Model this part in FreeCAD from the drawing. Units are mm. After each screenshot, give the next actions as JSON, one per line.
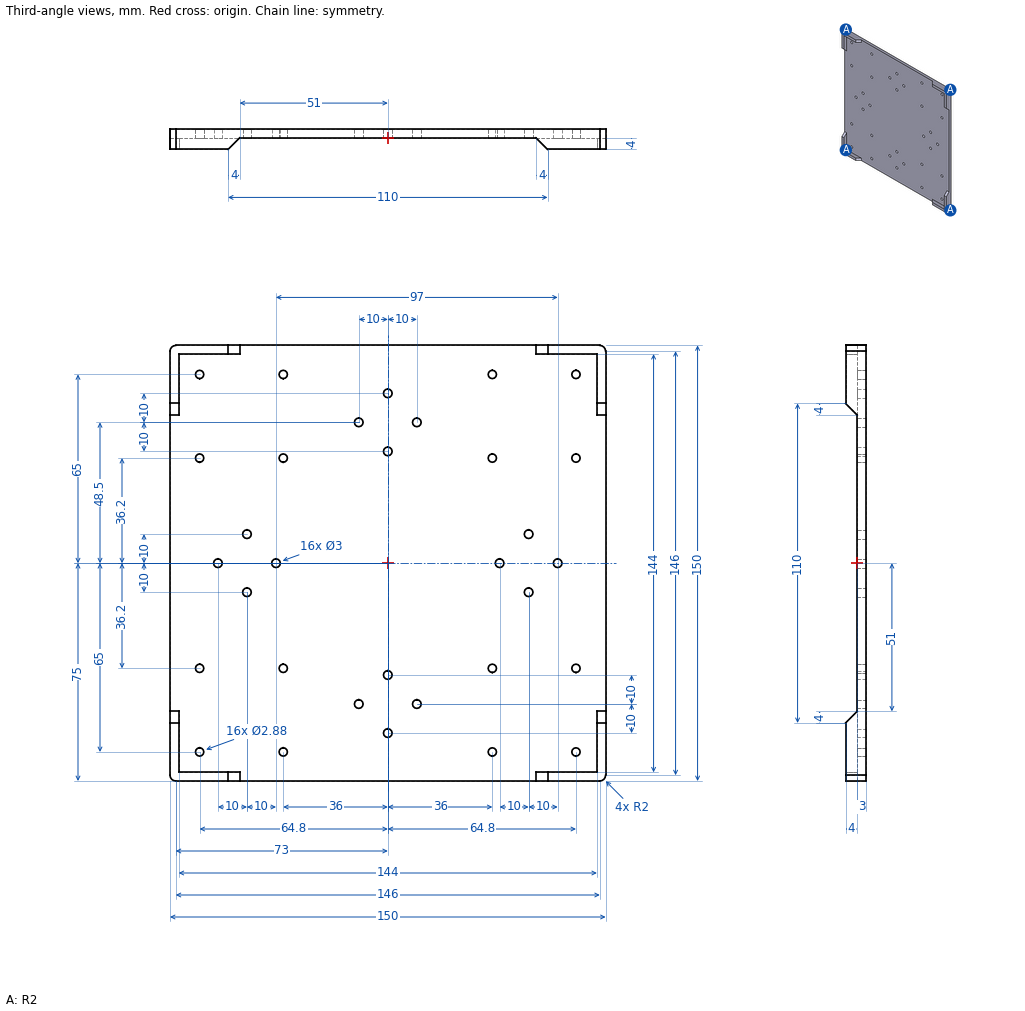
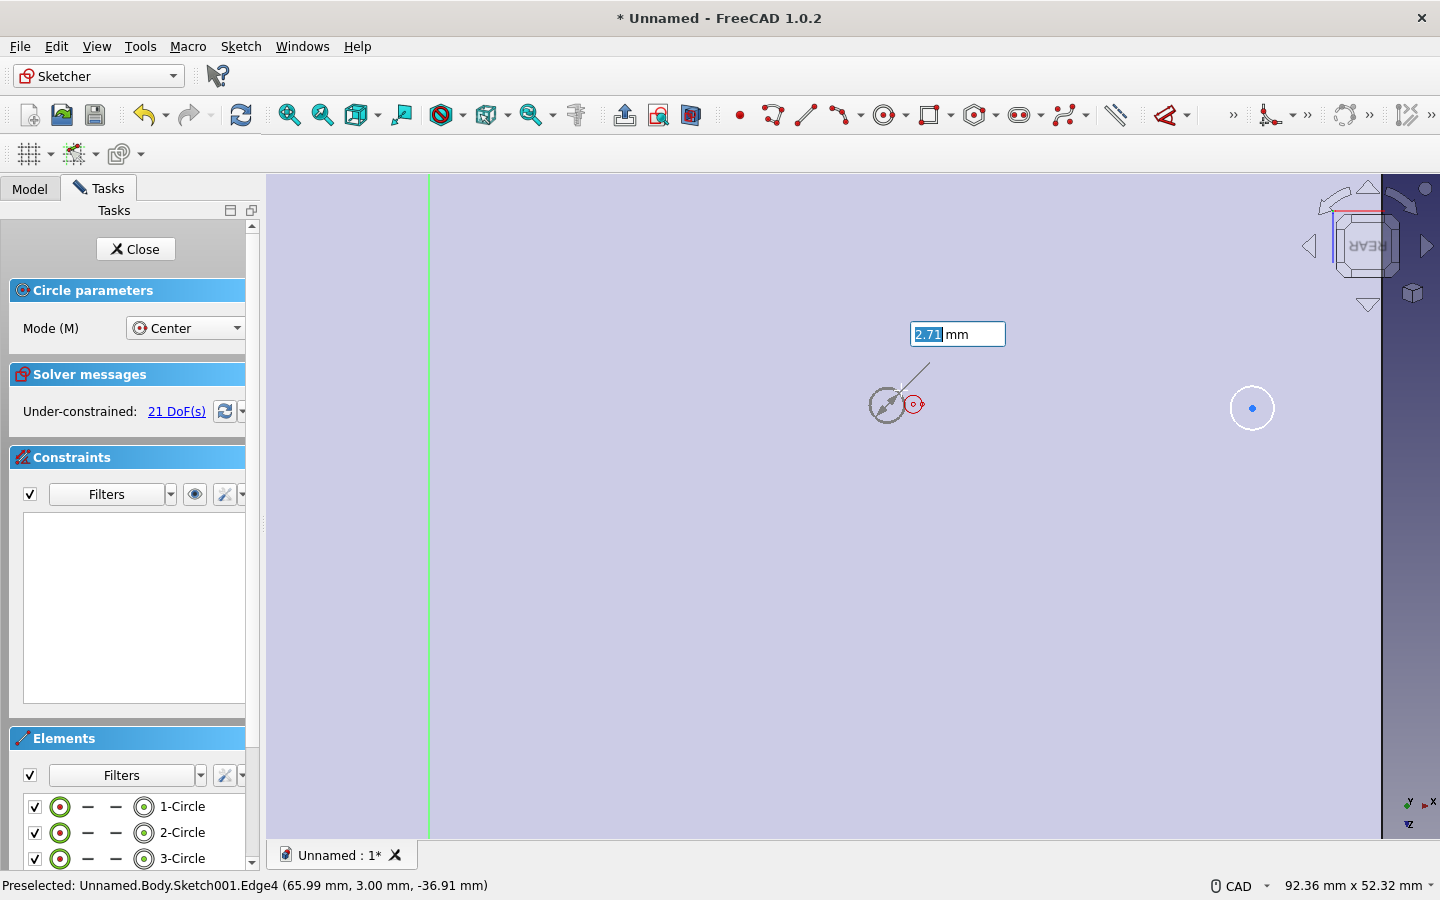
{"action": "left_click", "coordinate": [900, 389]}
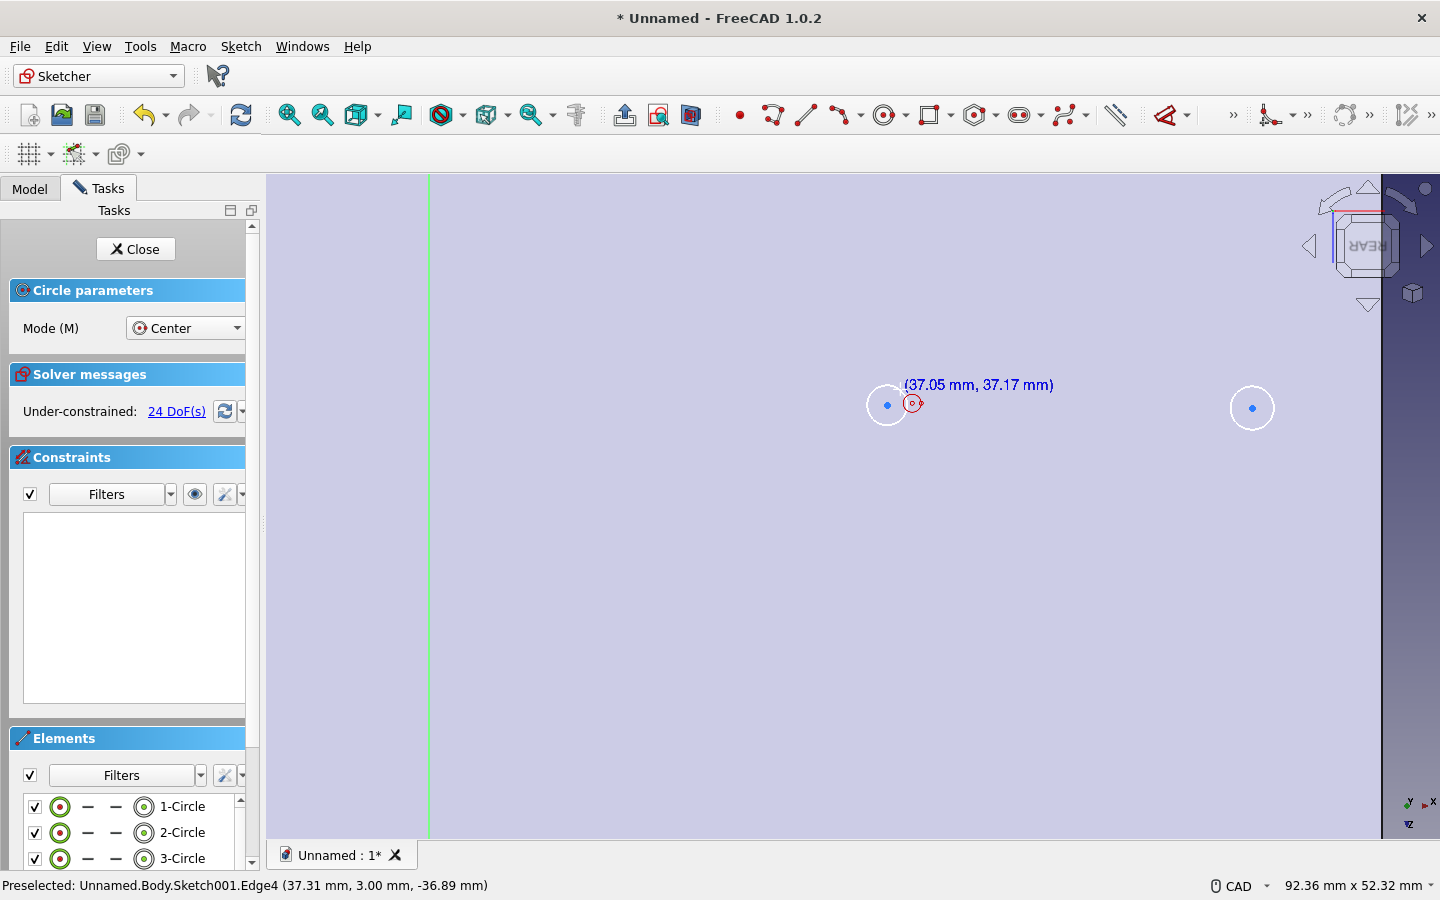
{"action": "scroll", "coordinate": [901, 390], "scroll_direction": "down", "scroll_amount": 7}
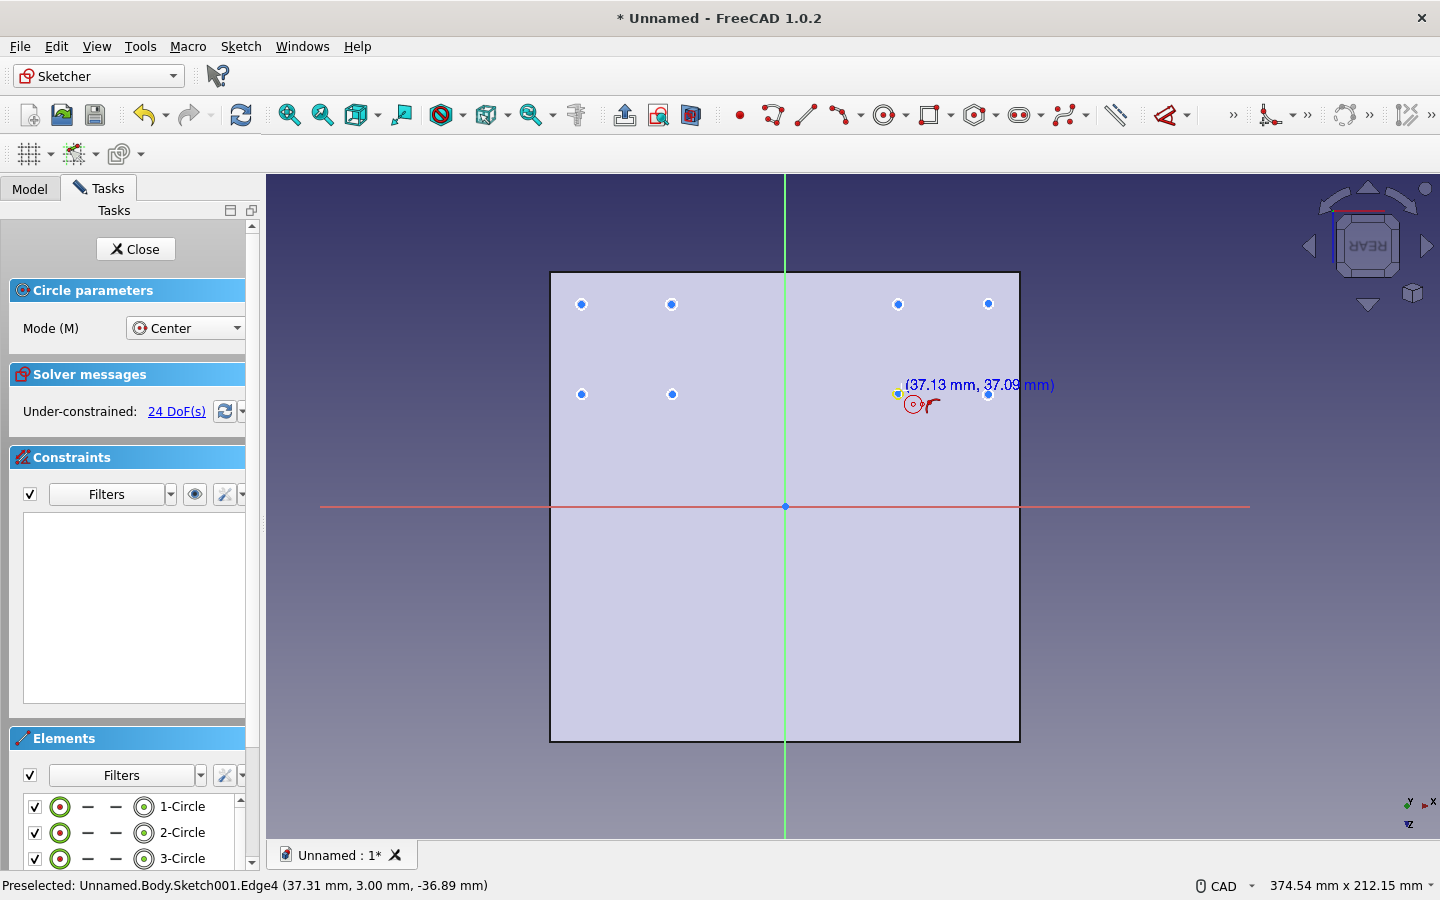
{"action": "scroll", "coordinate": [582, 620], "scroll_direction": "up", "scroll_amount": 9}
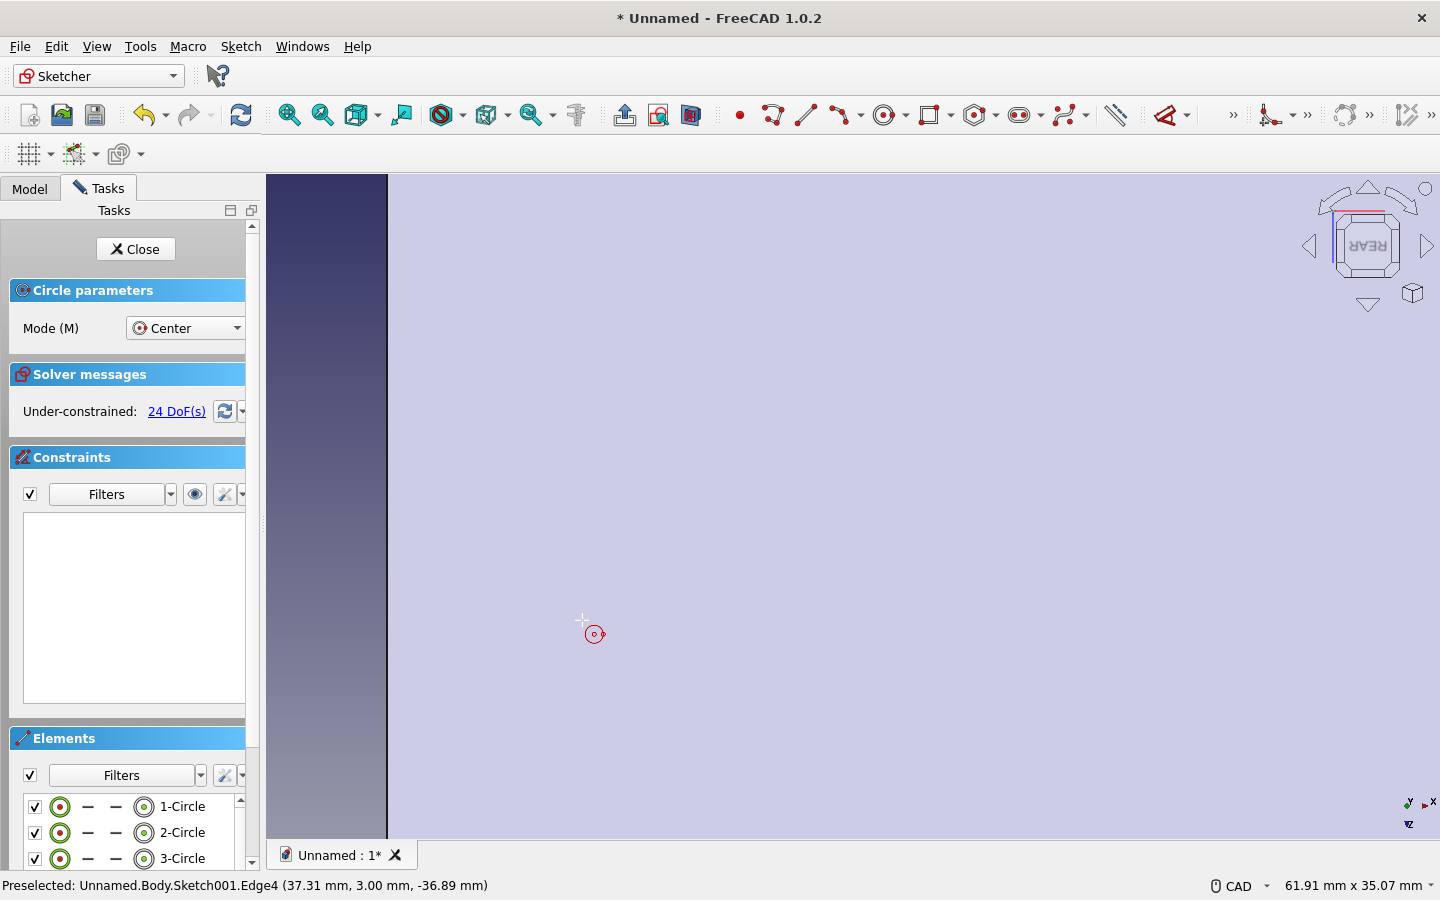
{"action": "scroll", "coordinate": [582, 620], "scroll_direction": "down", "scroll_amount": 9}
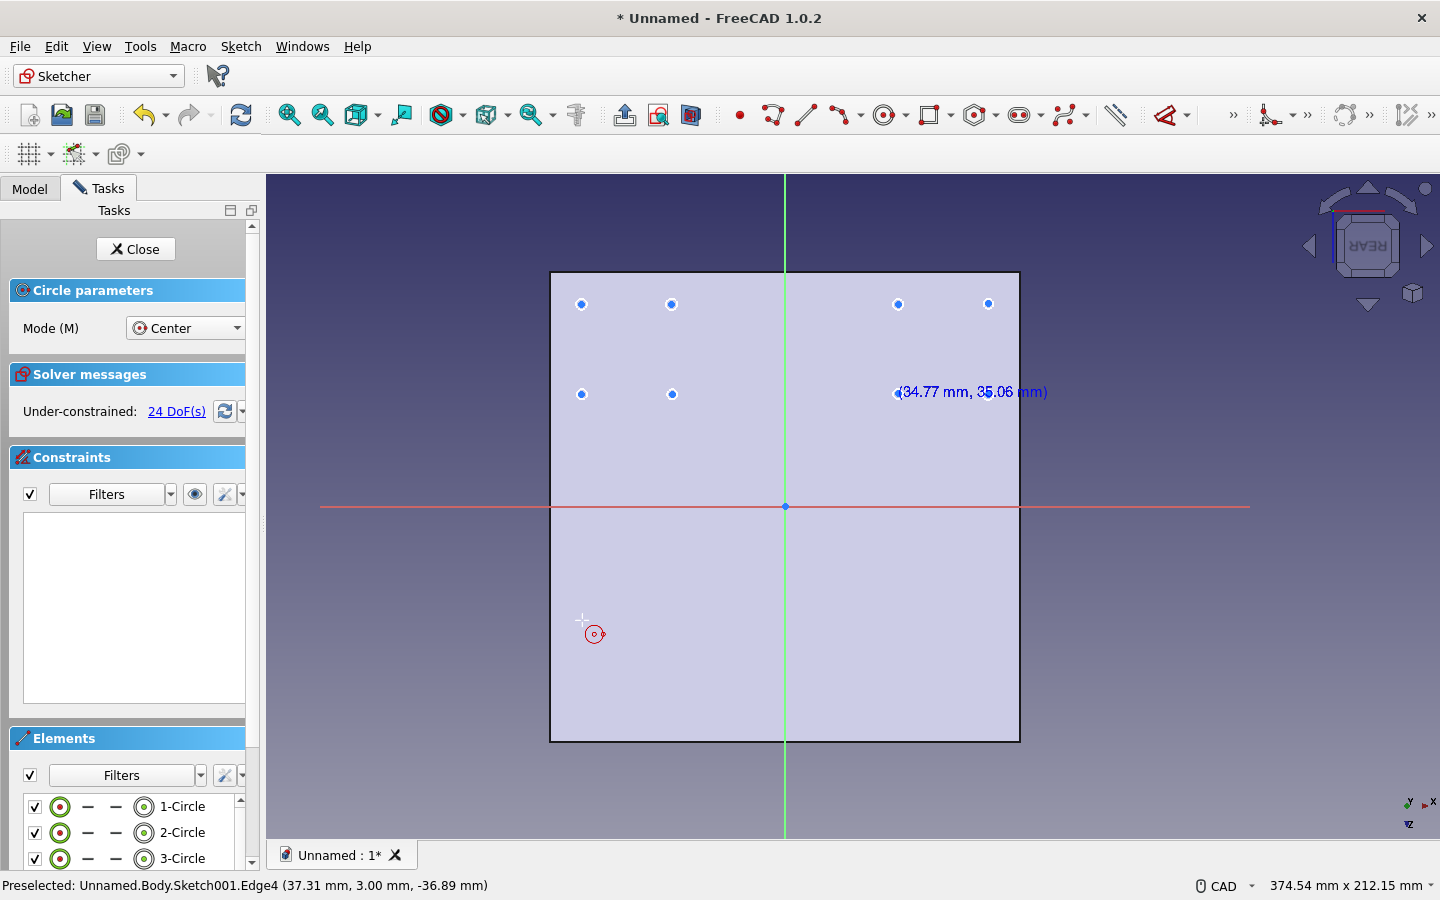
{"action": "left_click", "coordinate": [582, 620]}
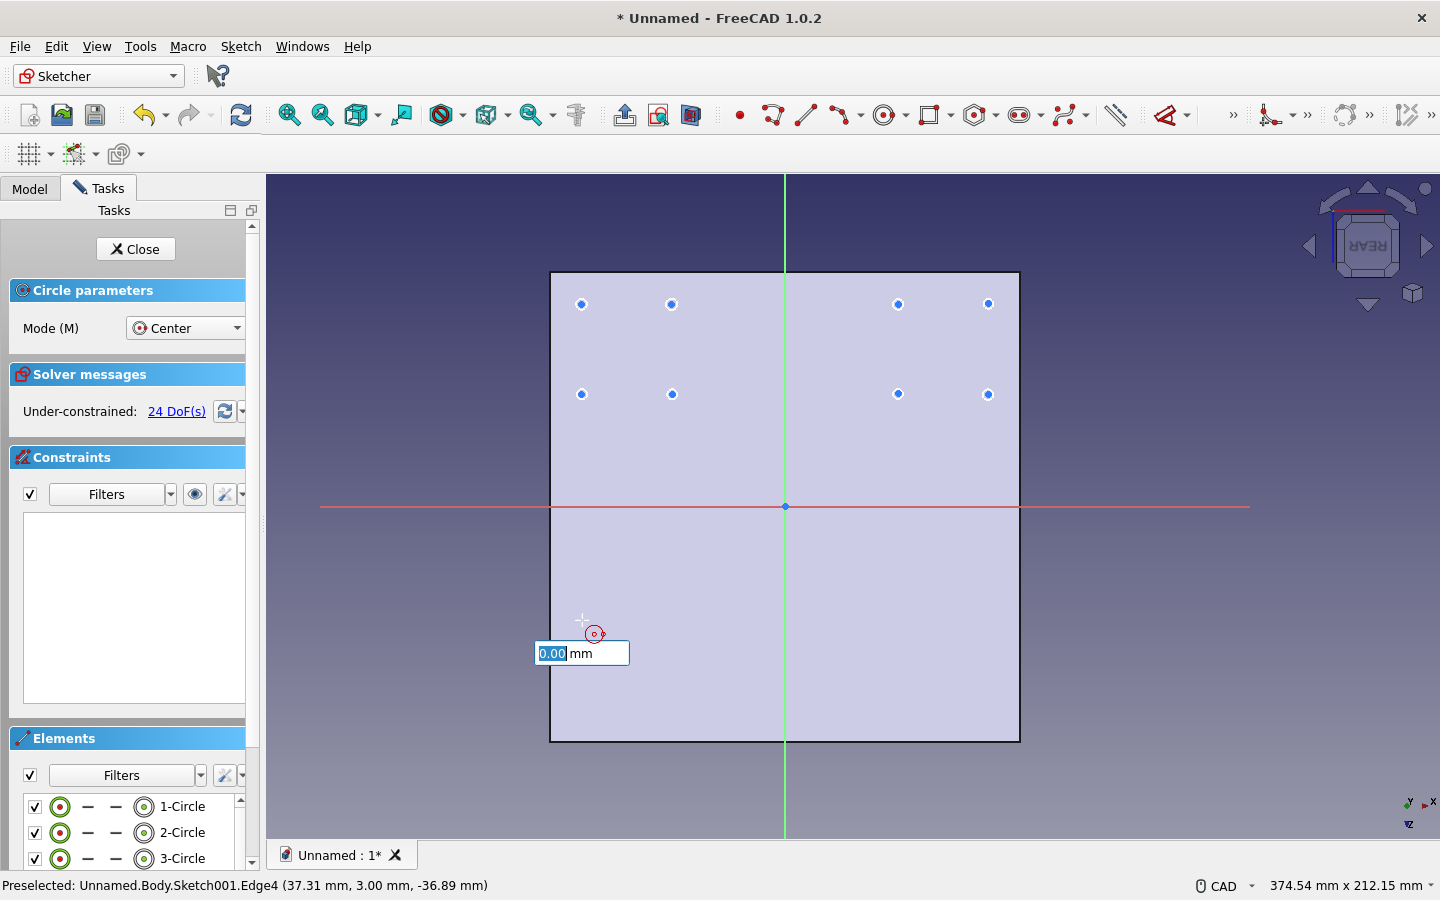
{"action": "scroll", "coordinate": [585, 617], "scroll_direction": "up", "scroll_amount": 7}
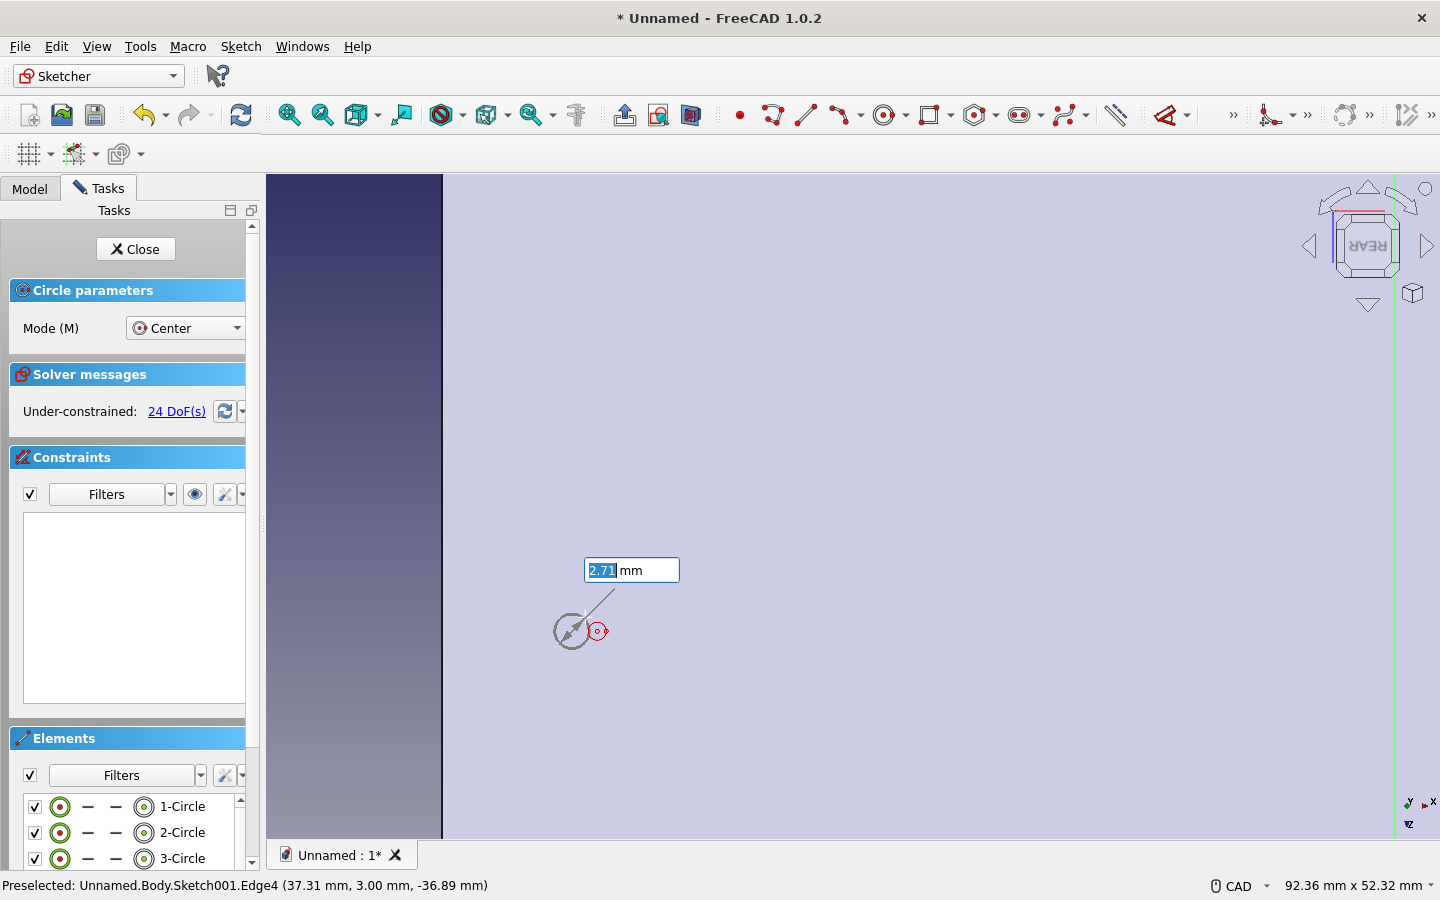
{"action": "left_click", "coordinate": [585, 615]}